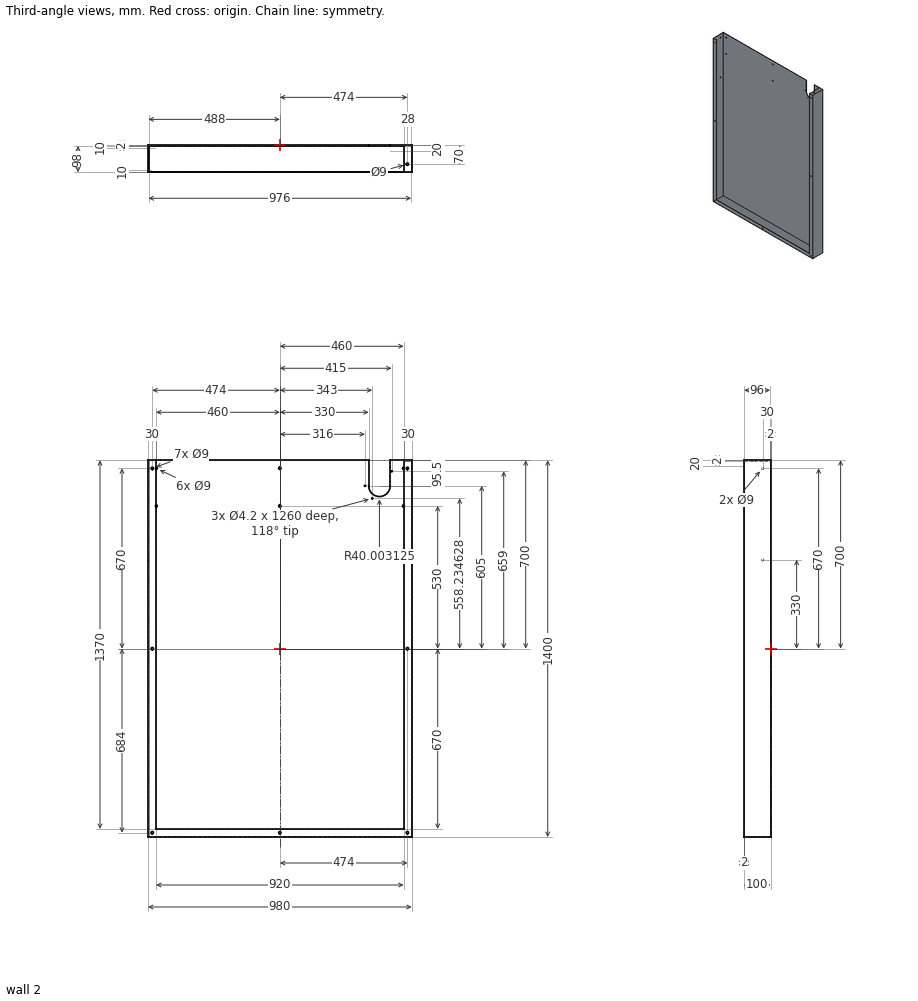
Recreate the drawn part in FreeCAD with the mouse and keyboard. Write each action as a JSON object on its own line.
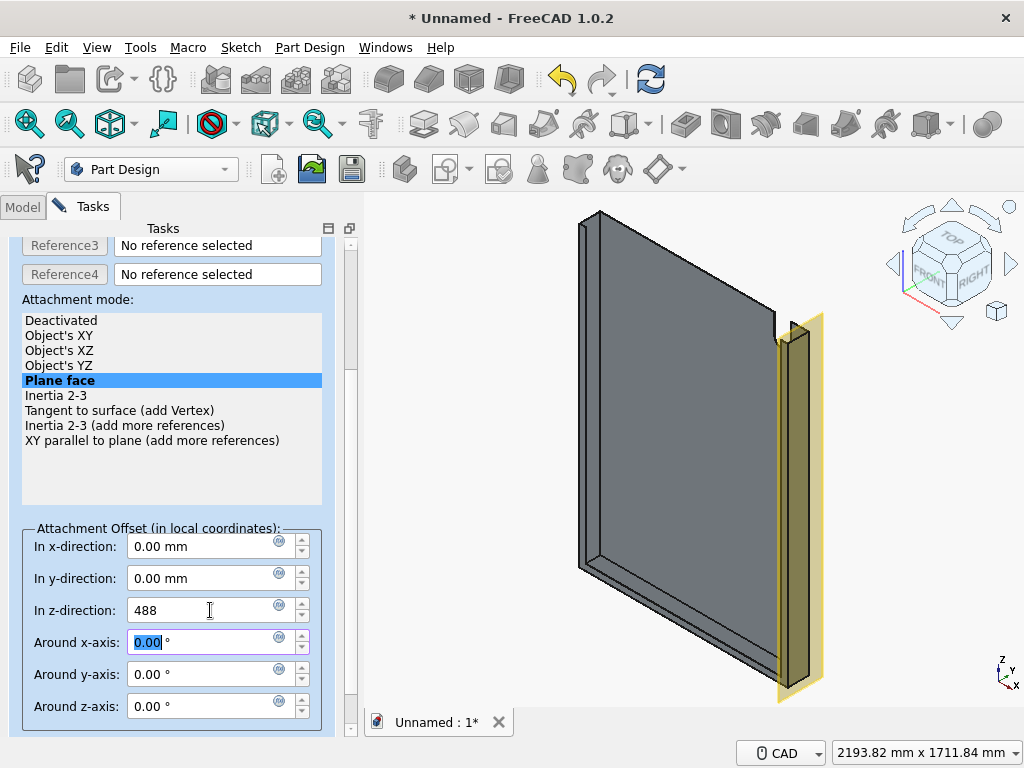
{"action": "scroll", "coordinate": [351, 487], "scroll_direction": "up", "scroll_amount": 4}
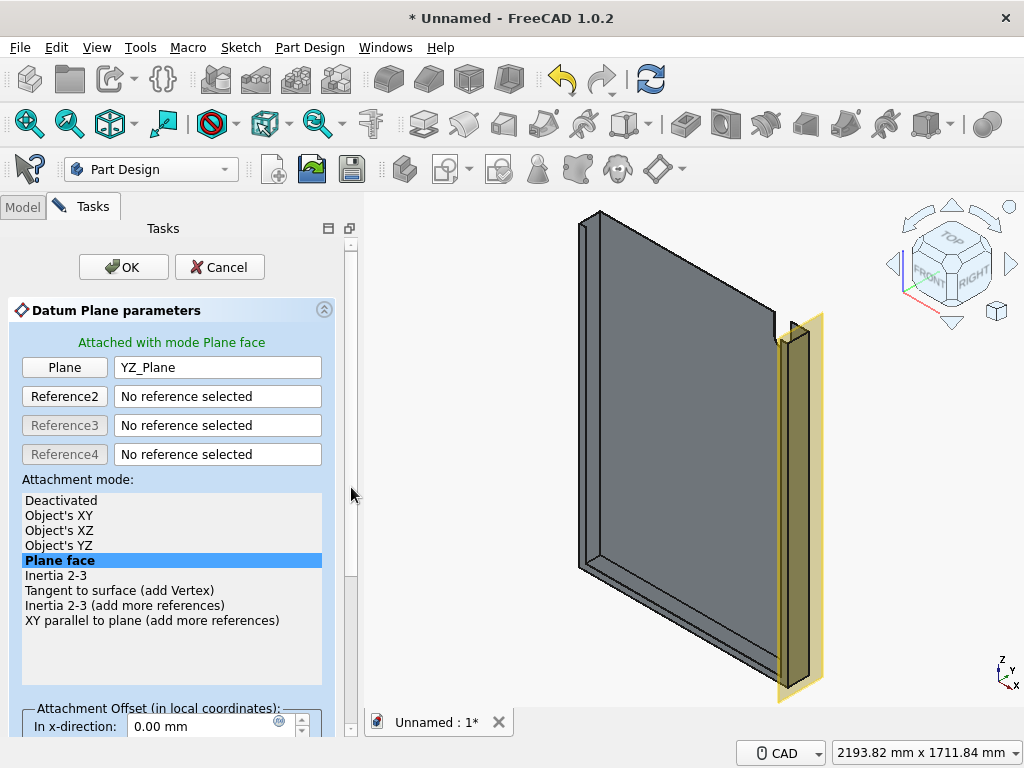
{"action": "left_click", "coordinate": [124, 267]}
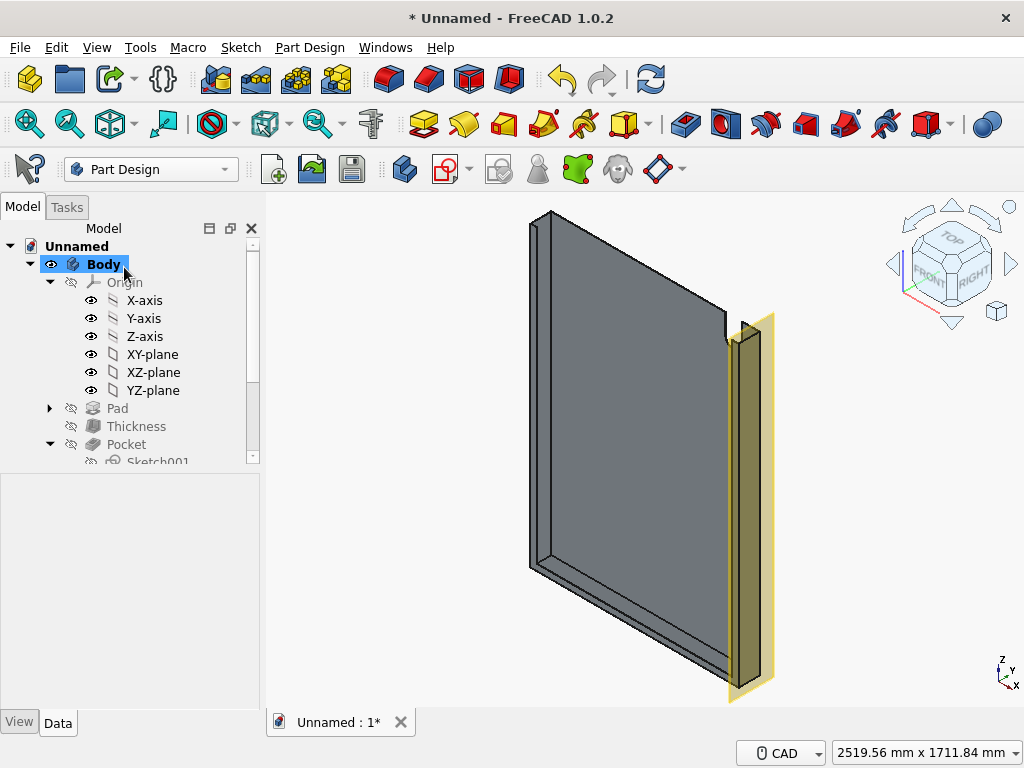
{"action": "scroll", "coordinate": [100, 350], "scroll_direction": "down", "scroll_amount": 3}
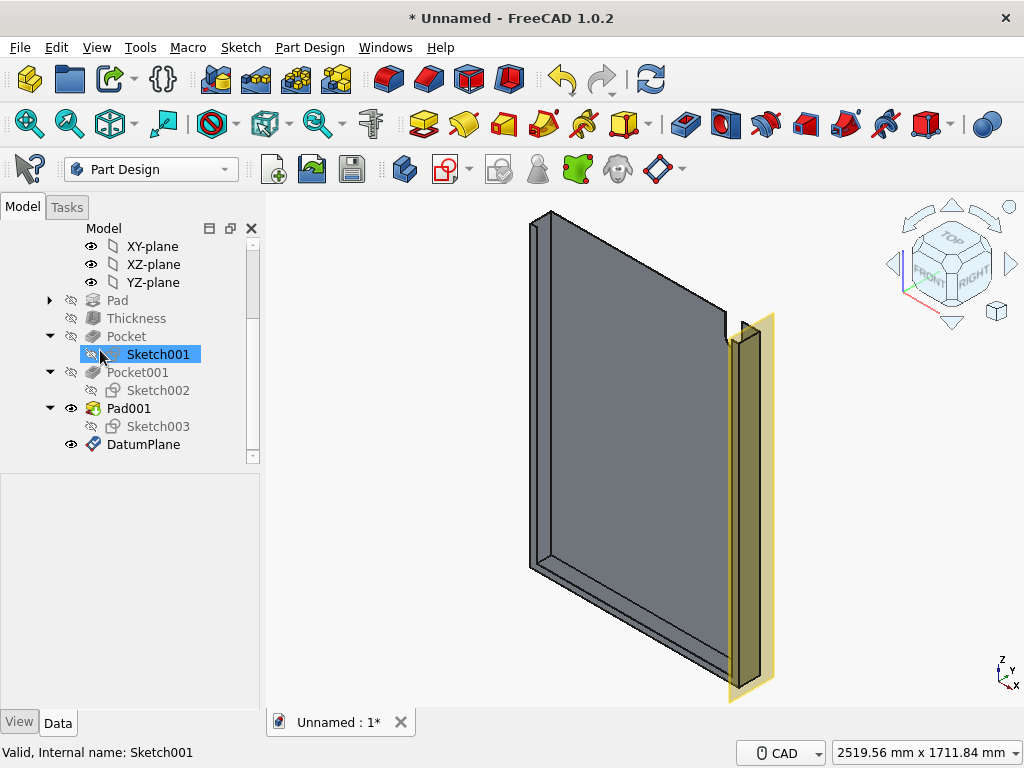
{"action": "left_click", "coordinate": [116, 444]}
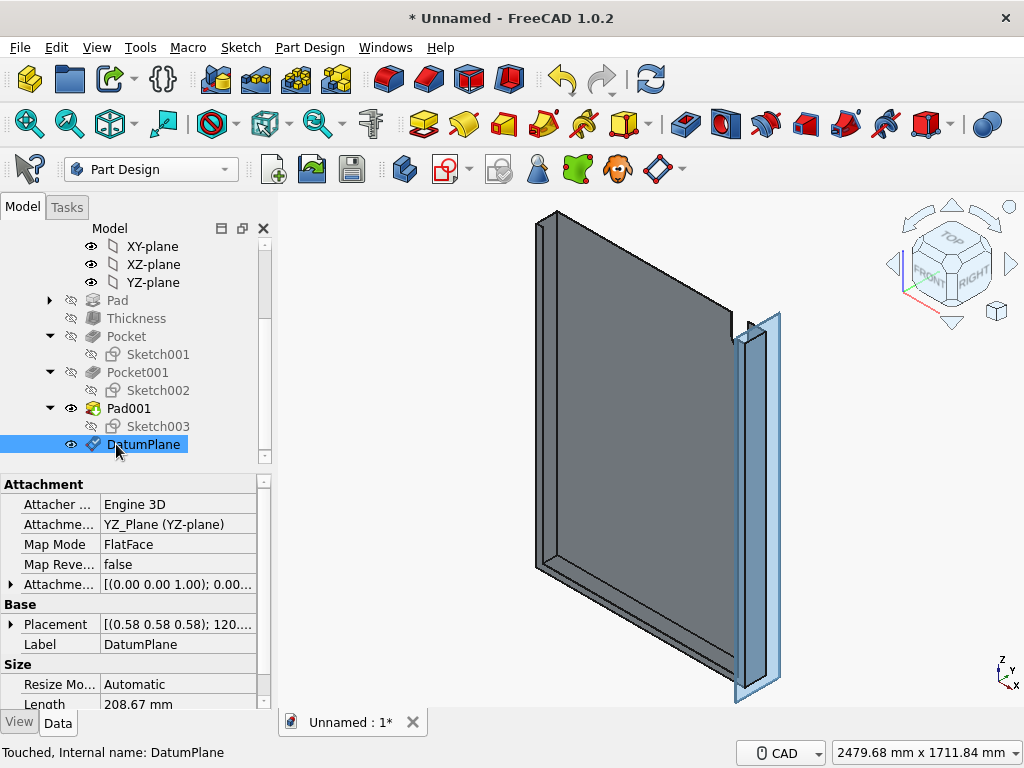
{"action": "left_click", "coordinate": [446, 170]}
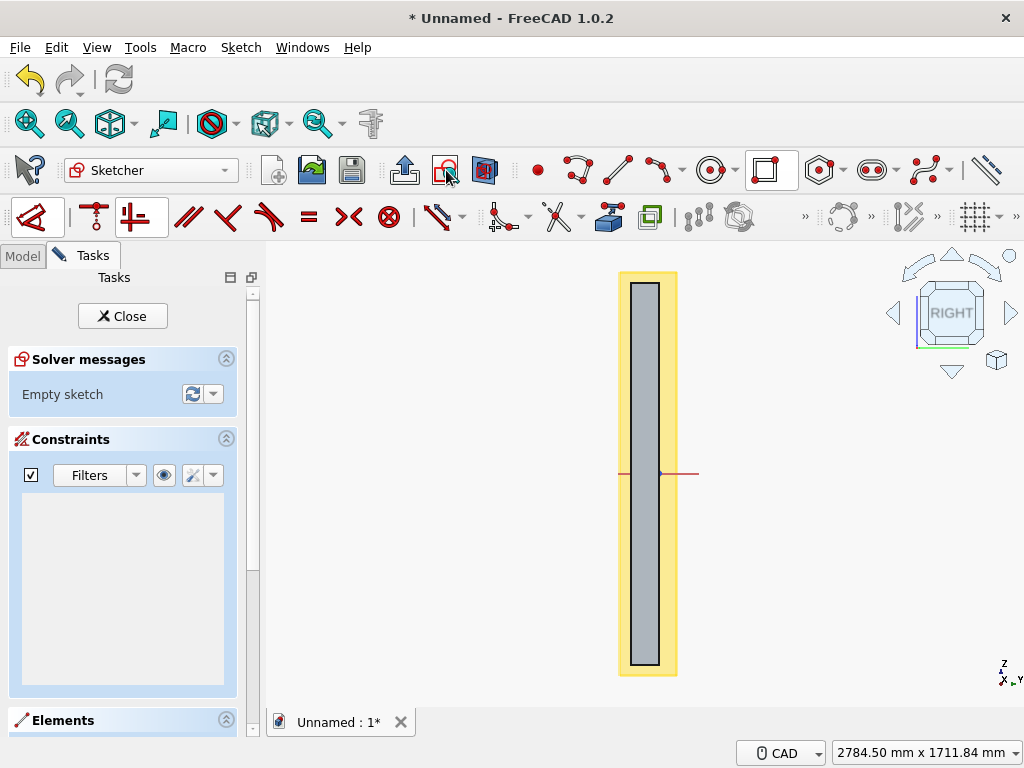
{"action": "left_click", "coordinate": [486, 170]}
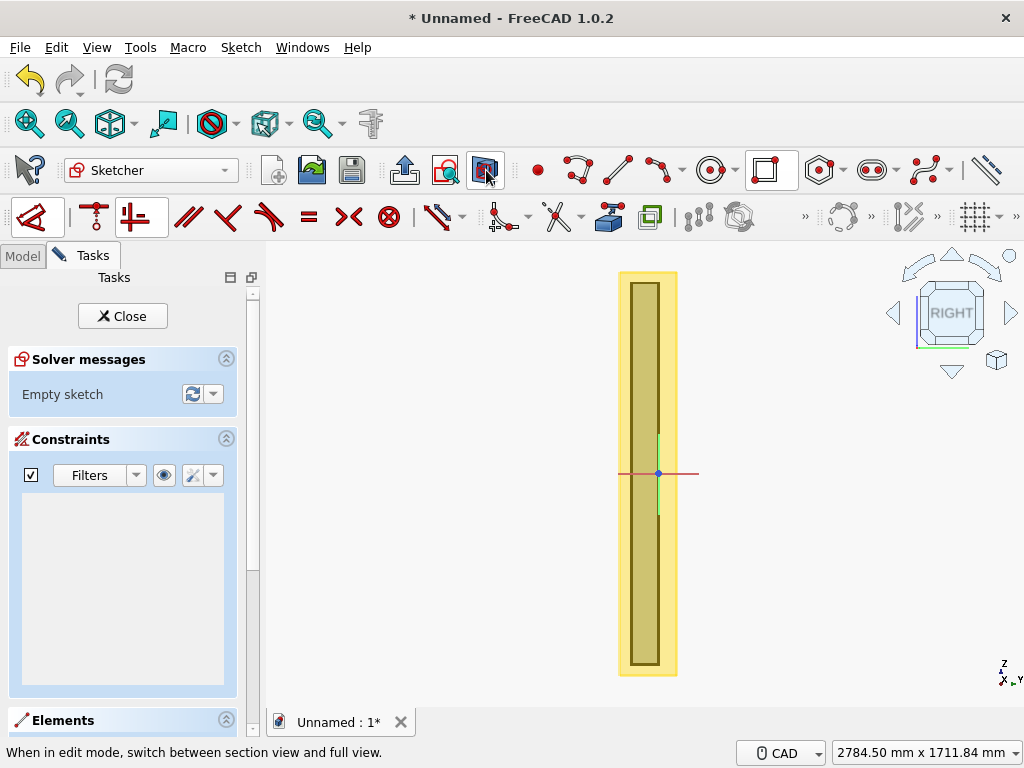
{"action": "scroll", "coordinate": [649, 271], "scroll_direction": "up", "scroll_amount": 14}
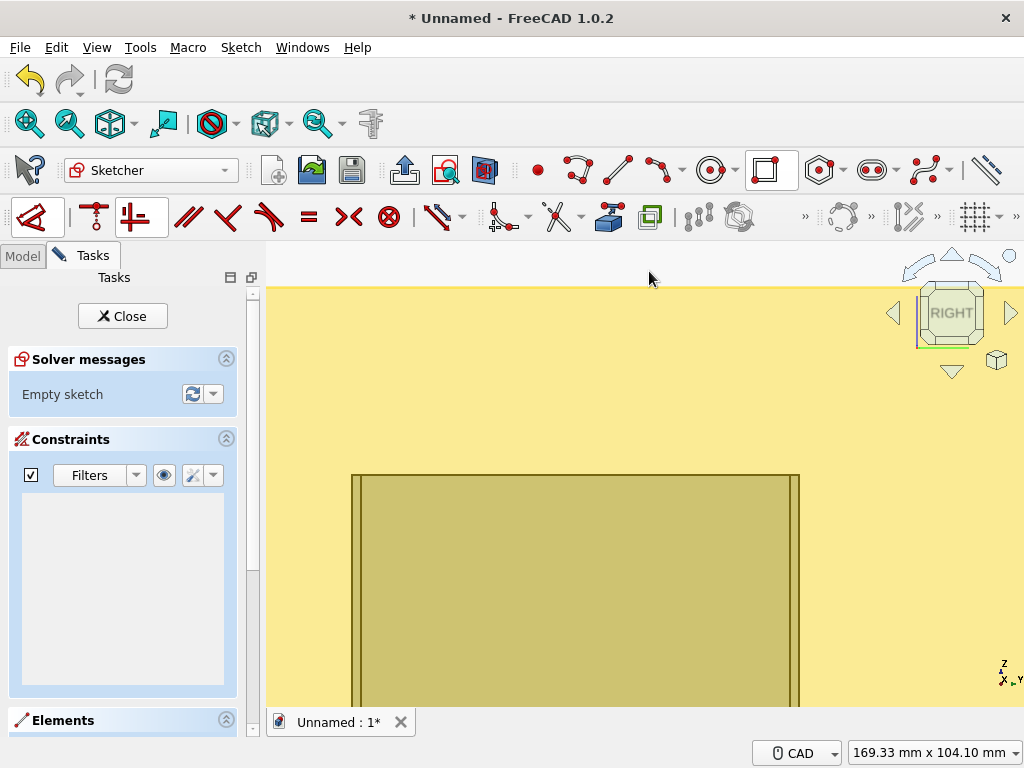
{"action": "left_click", "coordinate": [766, 170]}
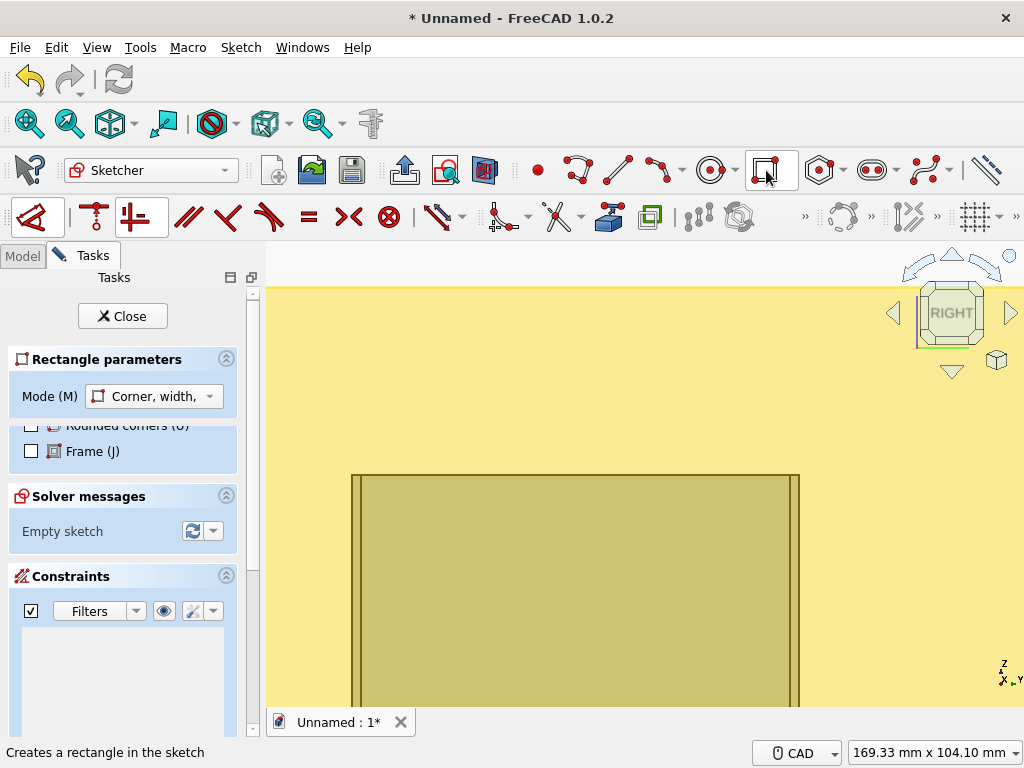
{"action": "scroll", "coordinate": [361, 475], "scroll_direction": "up", "scroll_amount": 3}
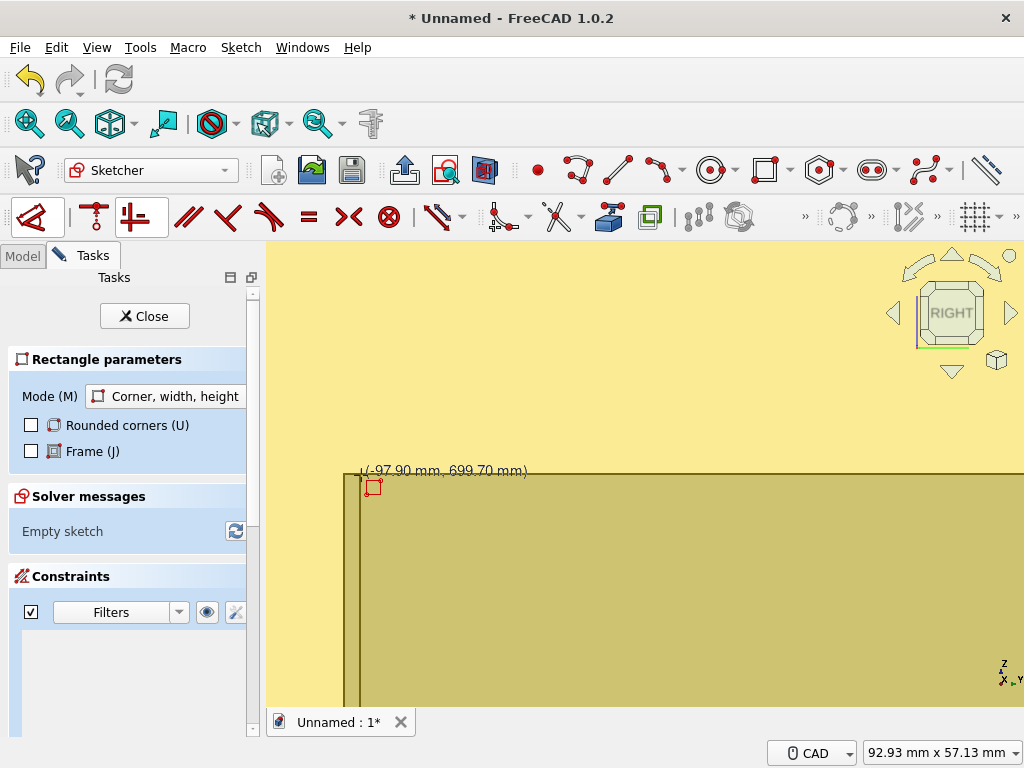
{"action": "left_click", "coordinate": [360, 474]}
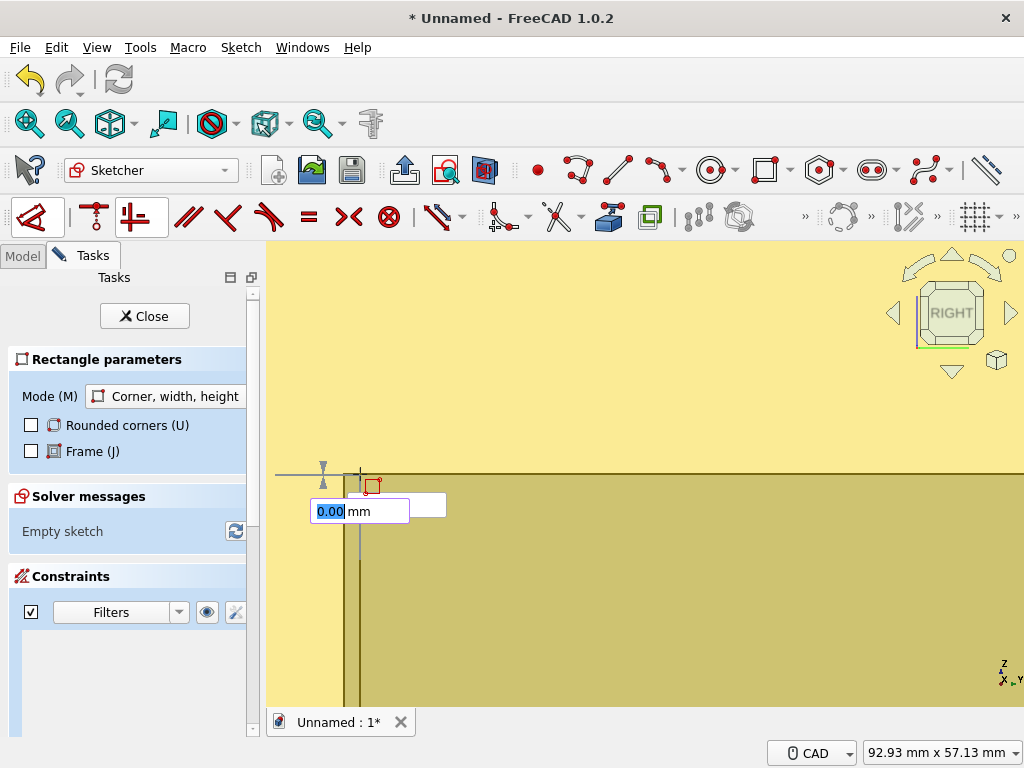
{"action": "scroll", "coordinate": [364, 464], "scroll_direction": "down", "scroll_amount": 3}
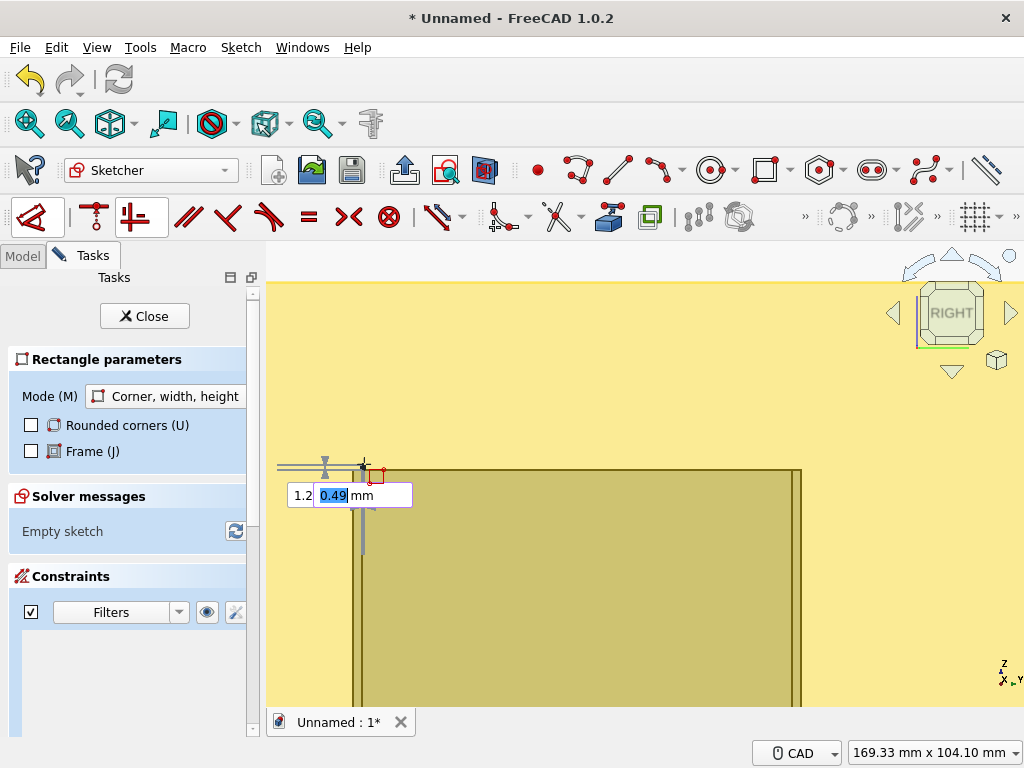
{"action": "scroll", "coordinate": [792, 479], "scroll_direction": "up", "scroll_amount": 3}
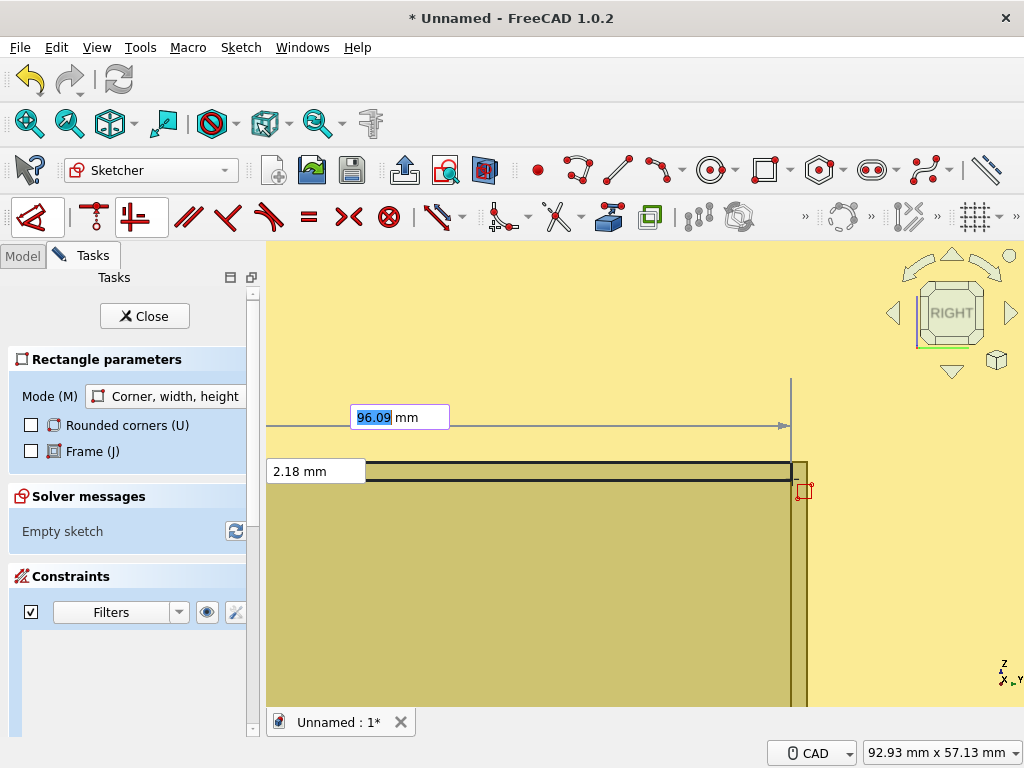
{"action": "left_click", "coordinate": [791, 478]}
{"action": "key", "text": "Escape"}